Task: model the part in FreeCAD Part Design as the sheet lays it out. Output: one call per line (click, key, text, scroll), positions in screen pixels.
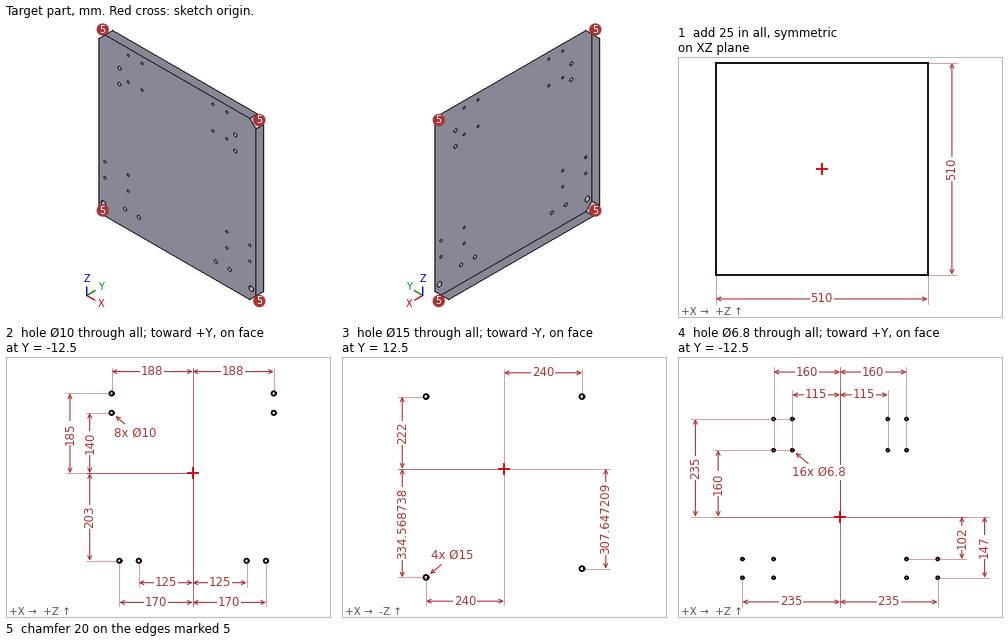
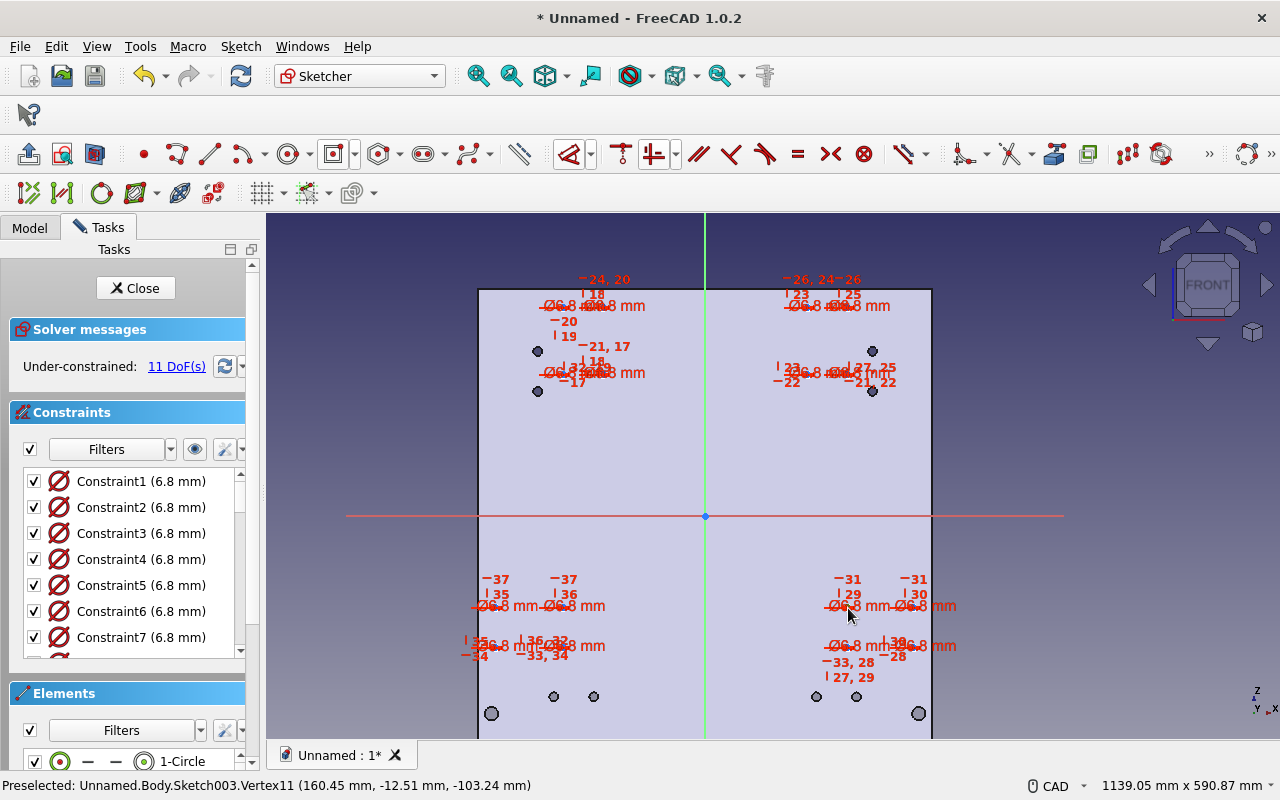
click(563, 608)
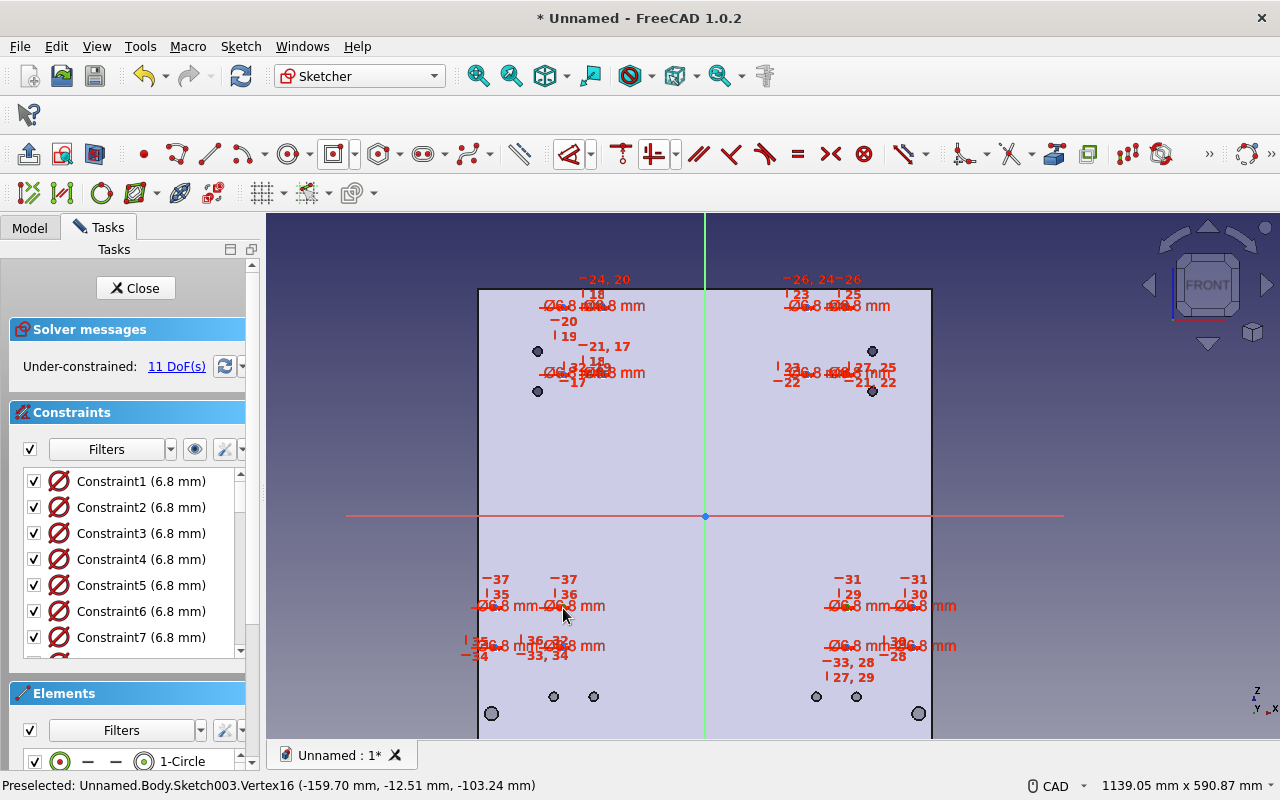
click(676, 154)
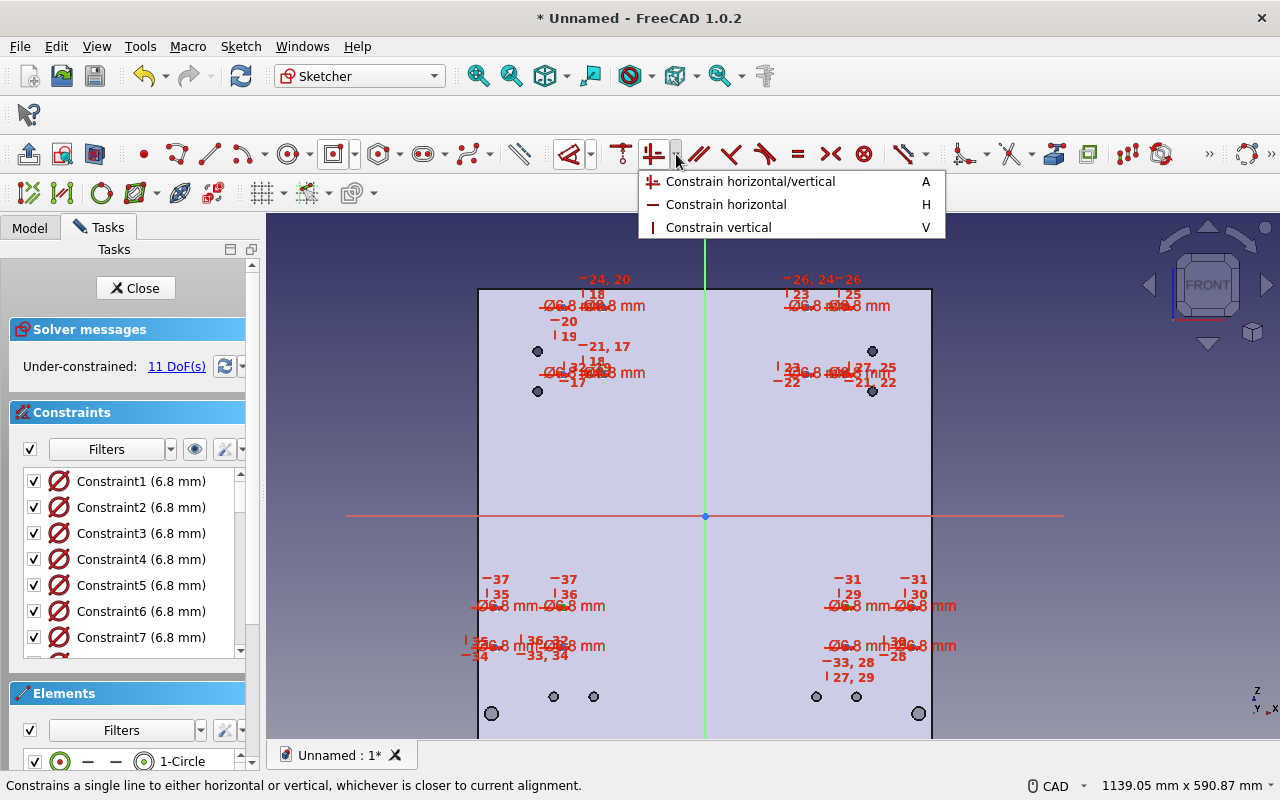
click(792, 204)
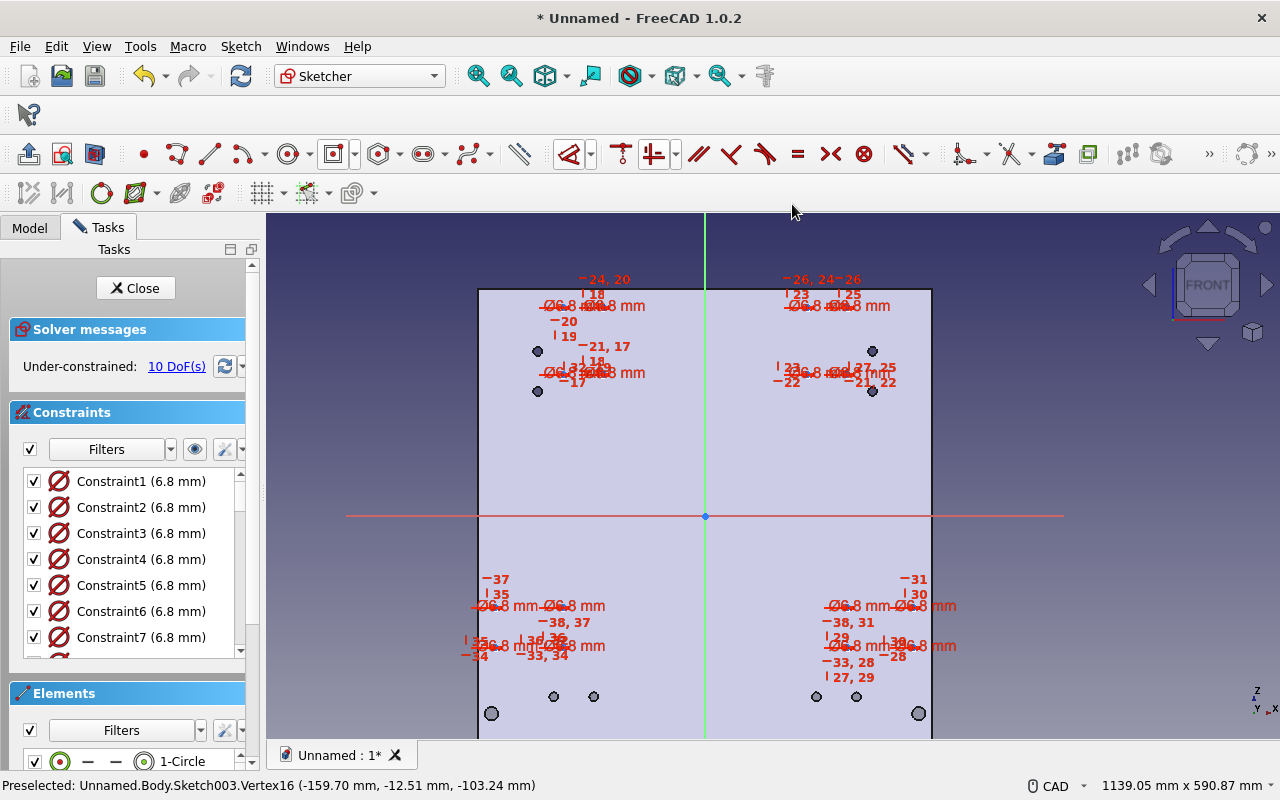
click(603, 375)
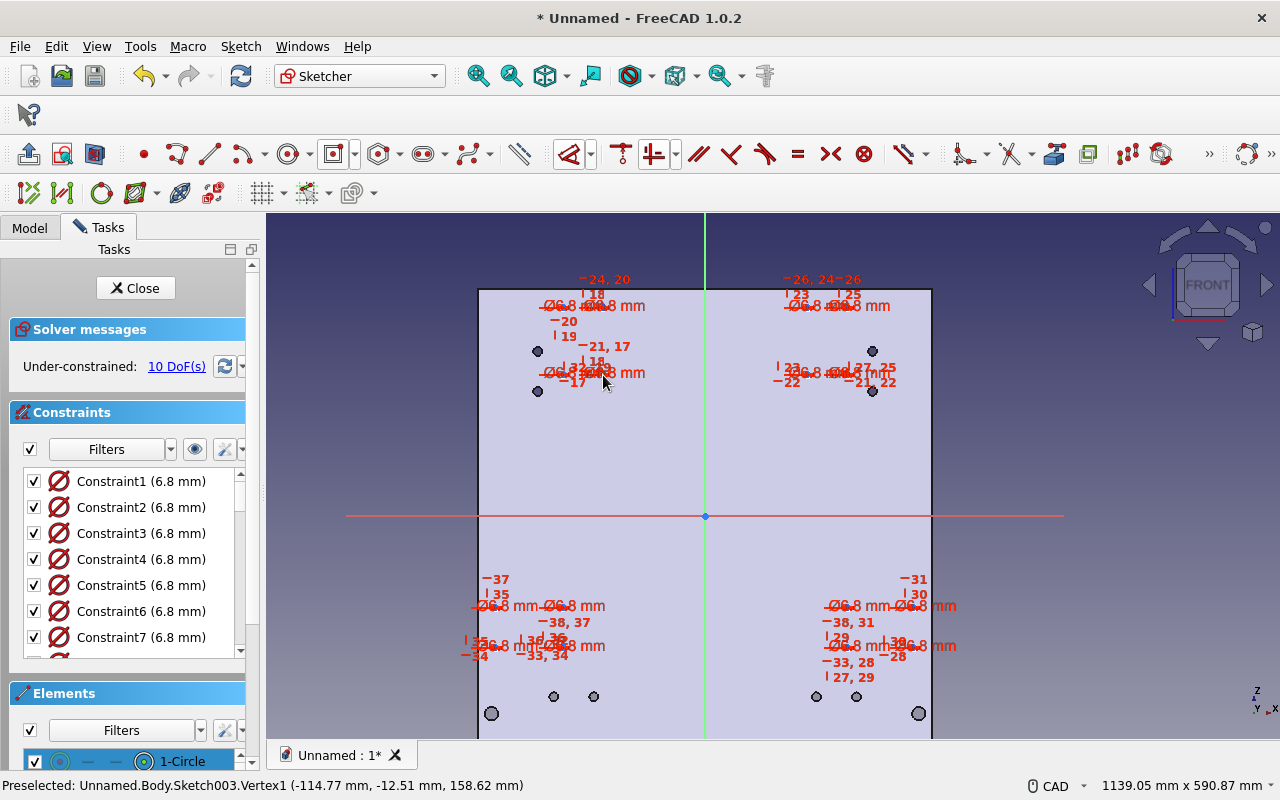
click(590, 154)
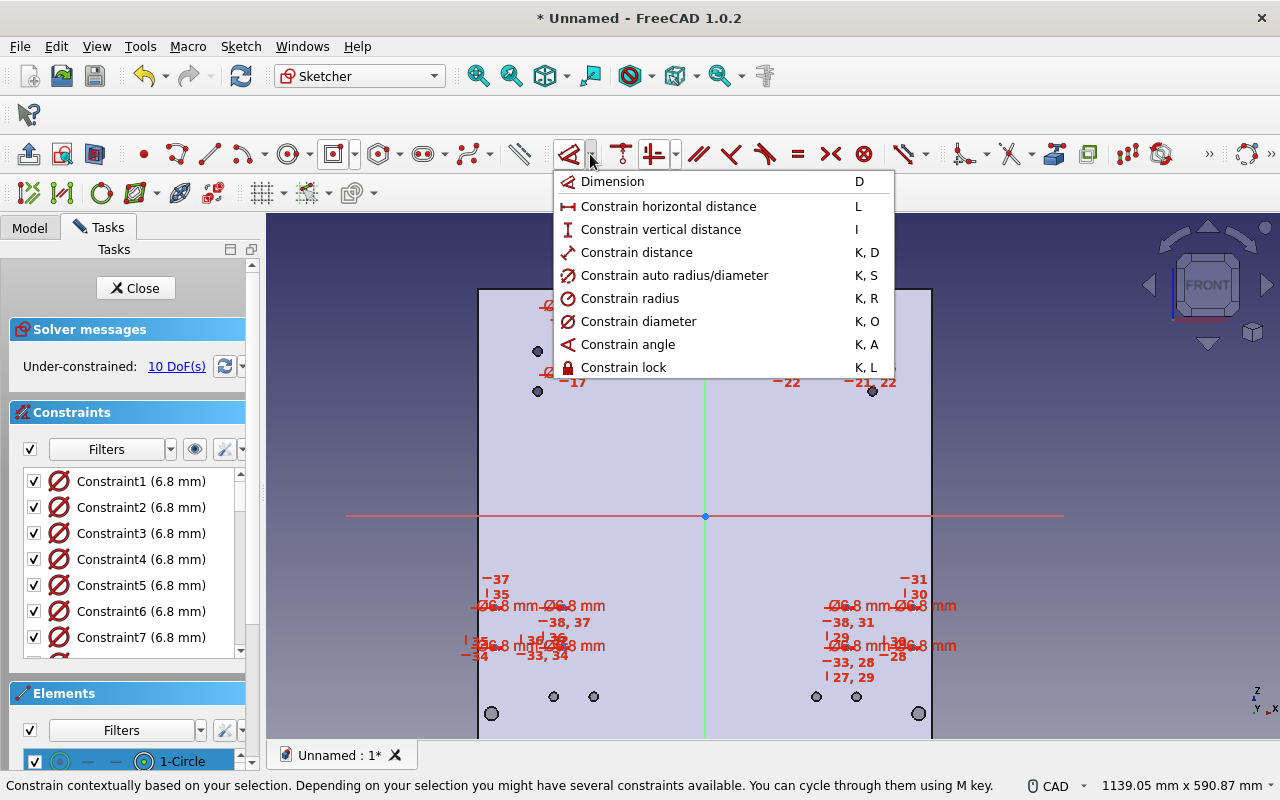
click(724, 206)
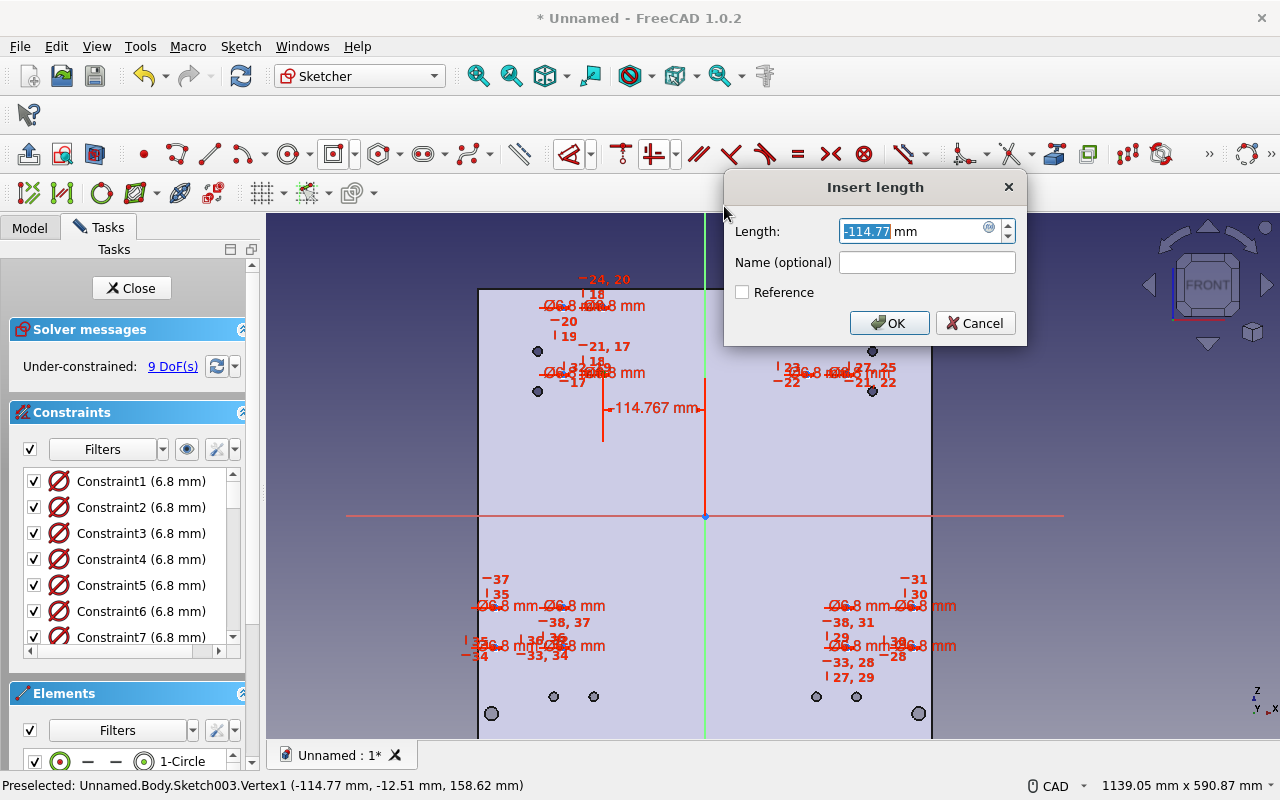
text(-115)
key(Return)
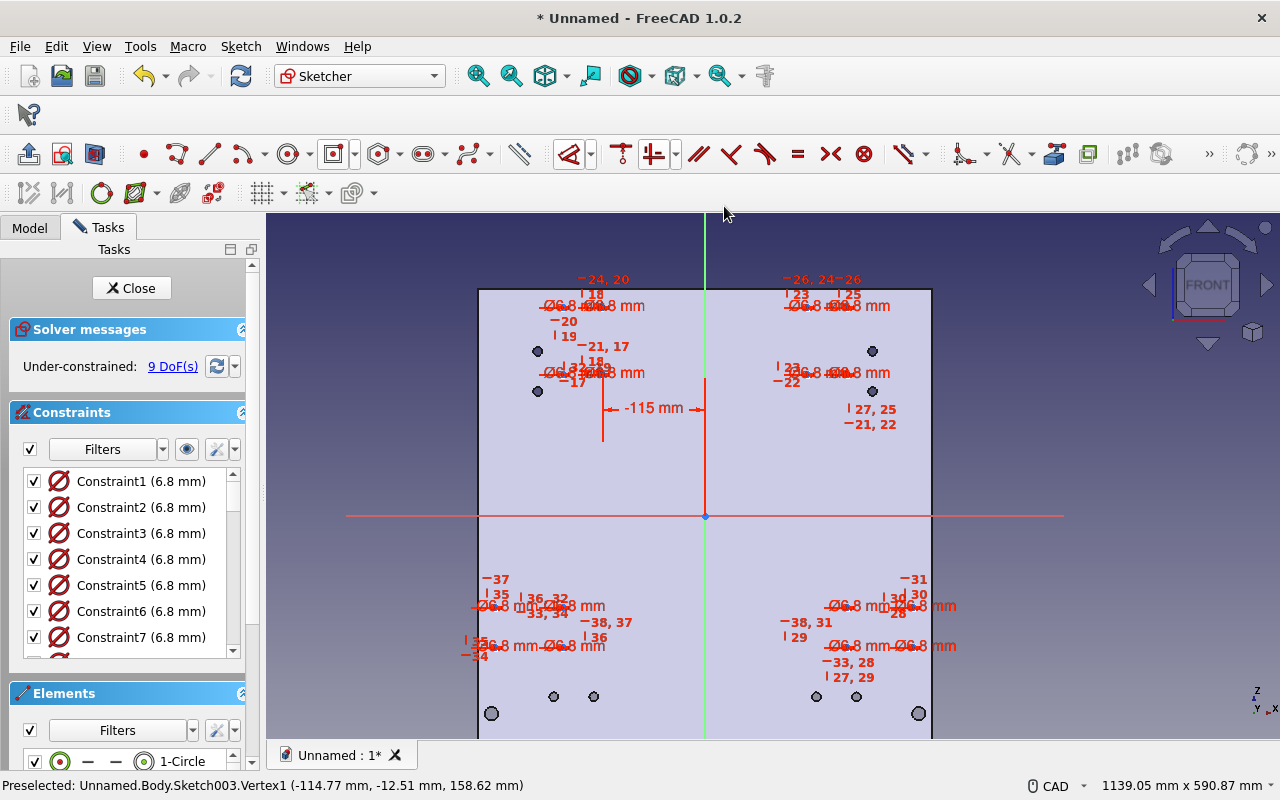
click(603, 375)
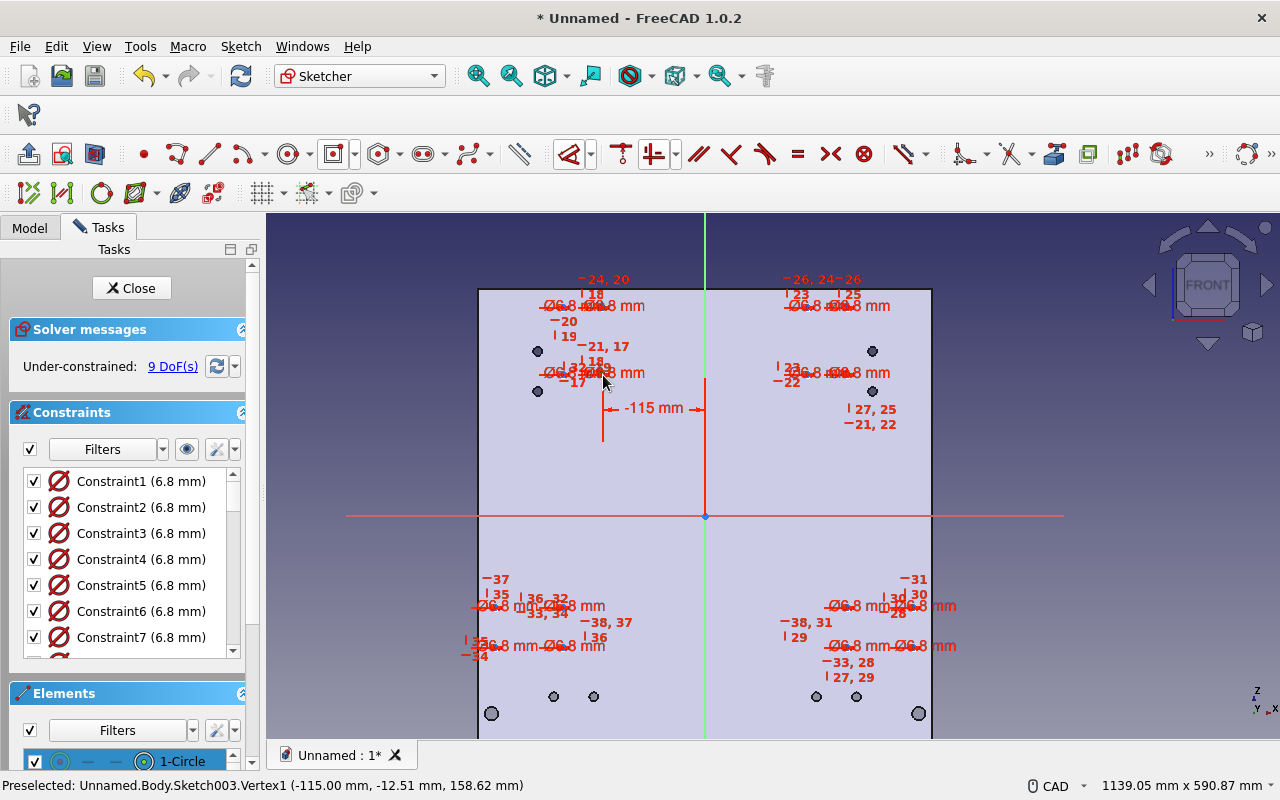
click(590, 154)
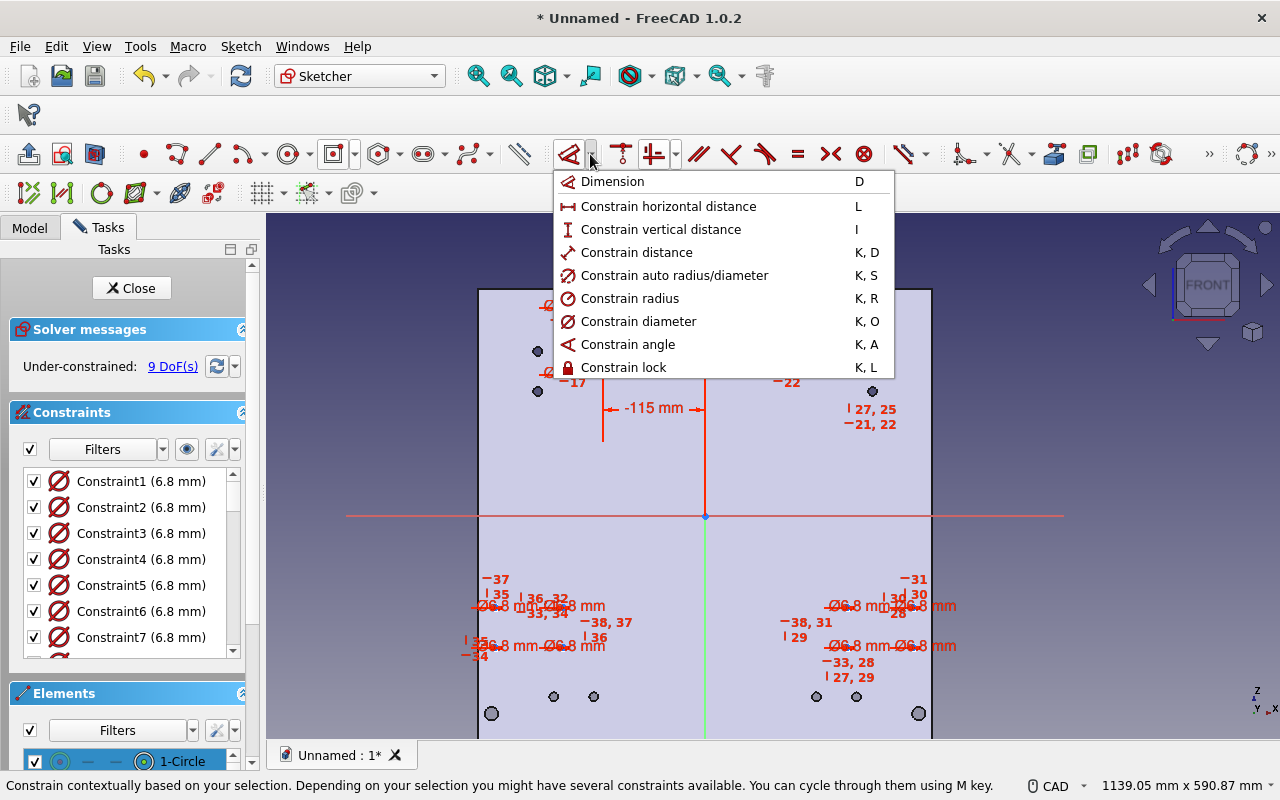
click(724, 230)